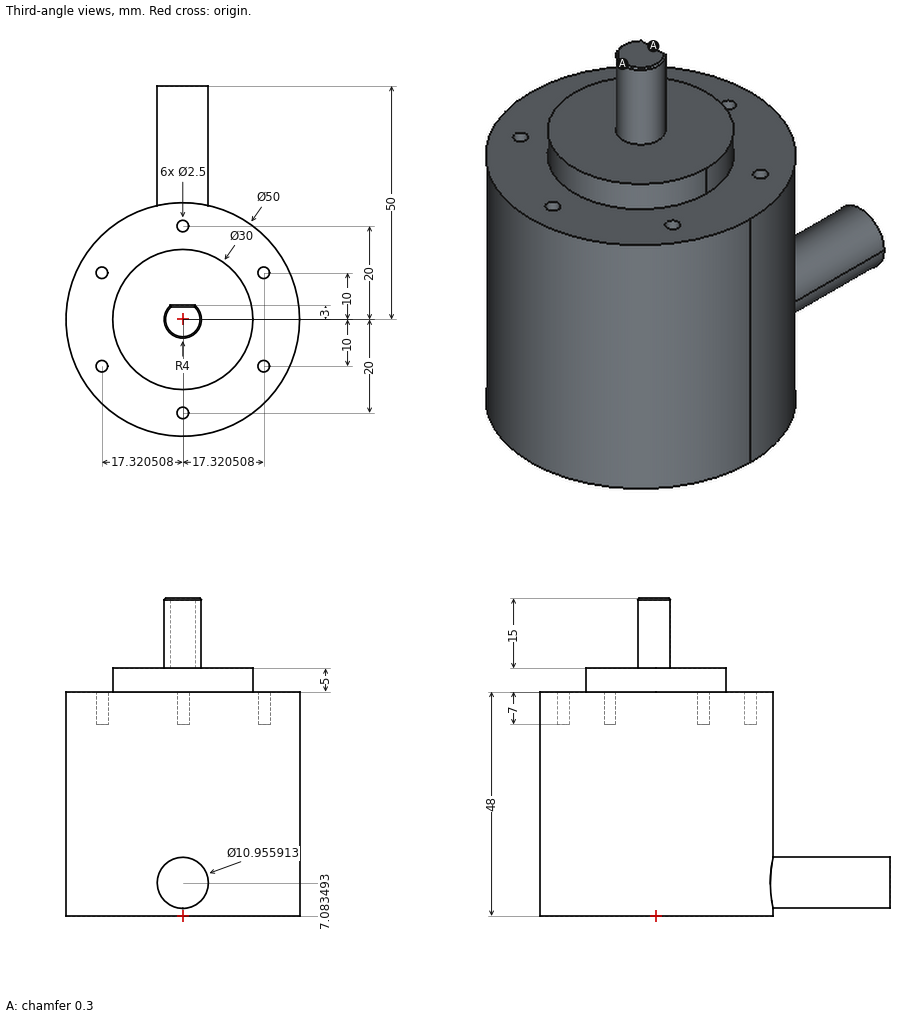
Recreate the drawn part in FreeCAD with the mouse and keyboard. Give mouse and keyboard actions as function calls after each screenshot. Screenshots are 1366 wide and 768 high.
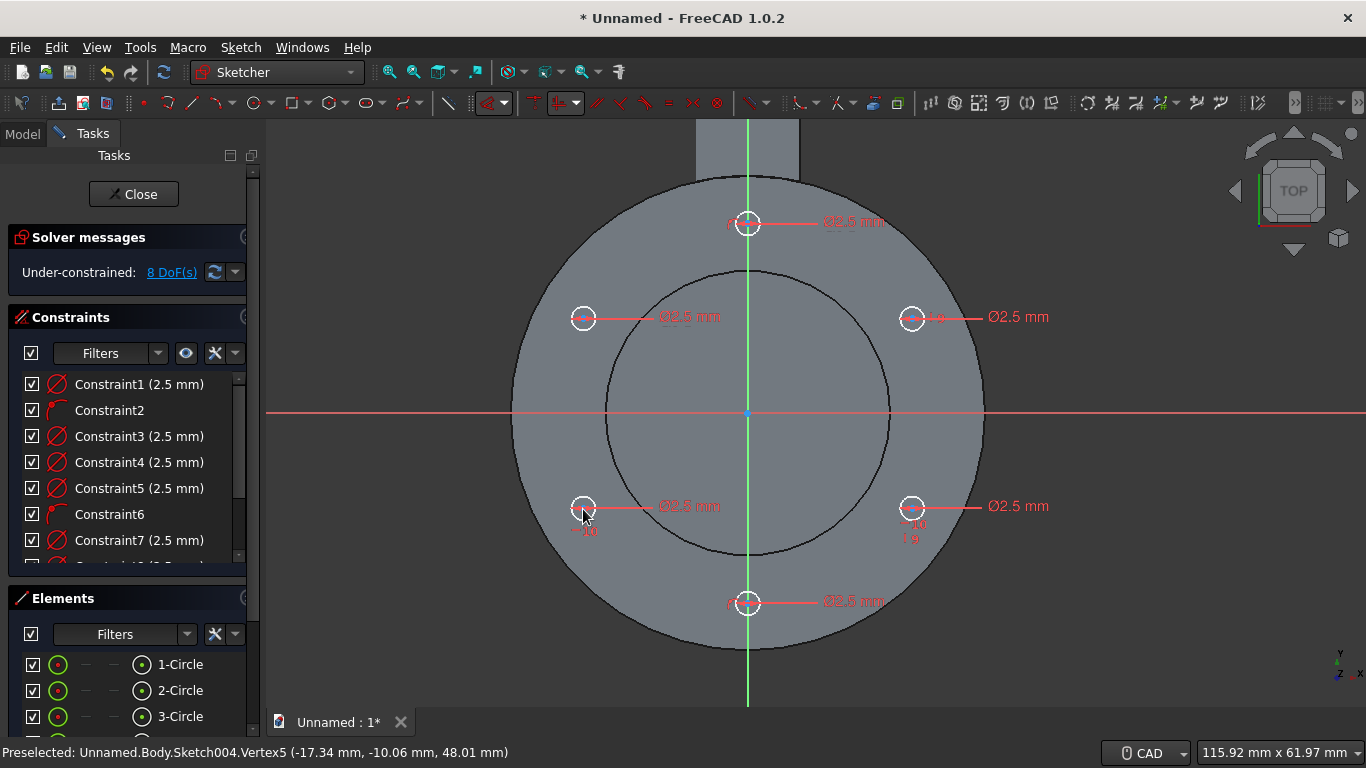
click(583, 508)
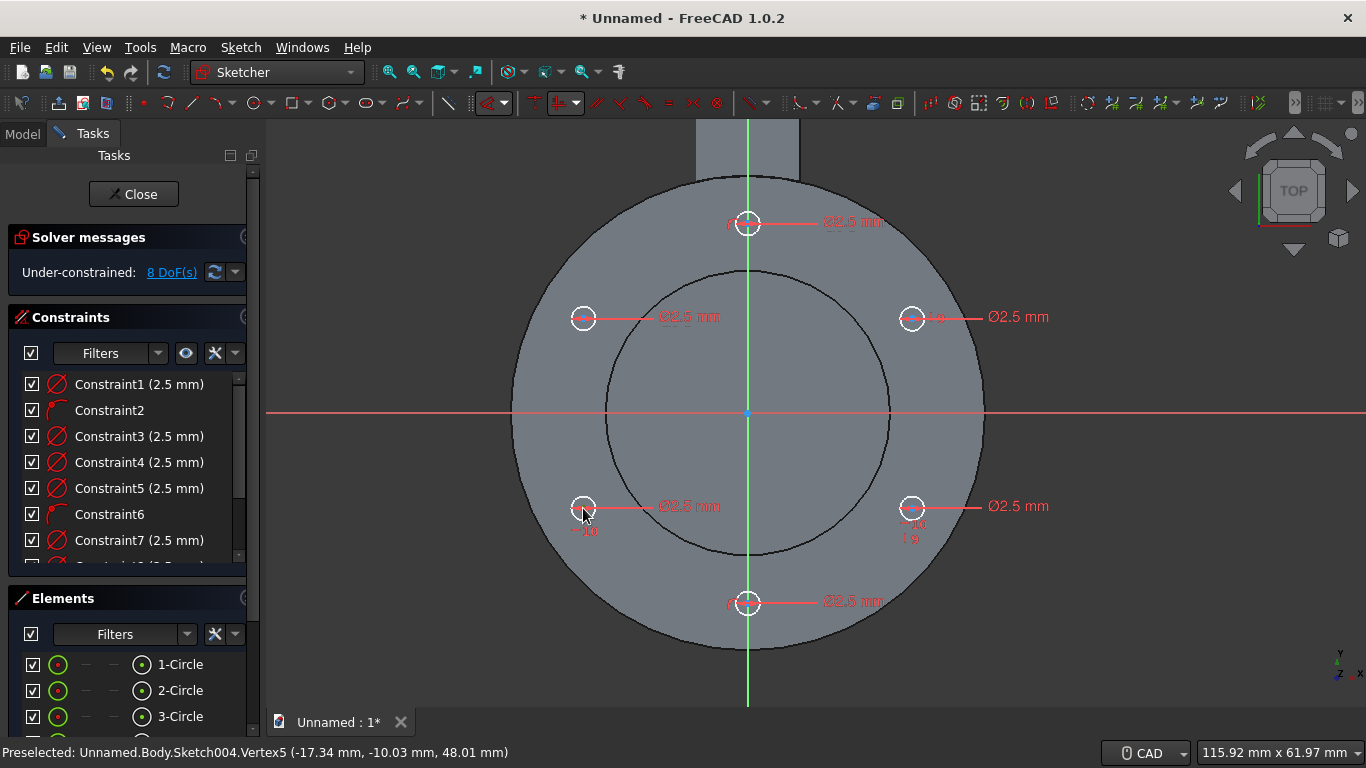
click(584, 319)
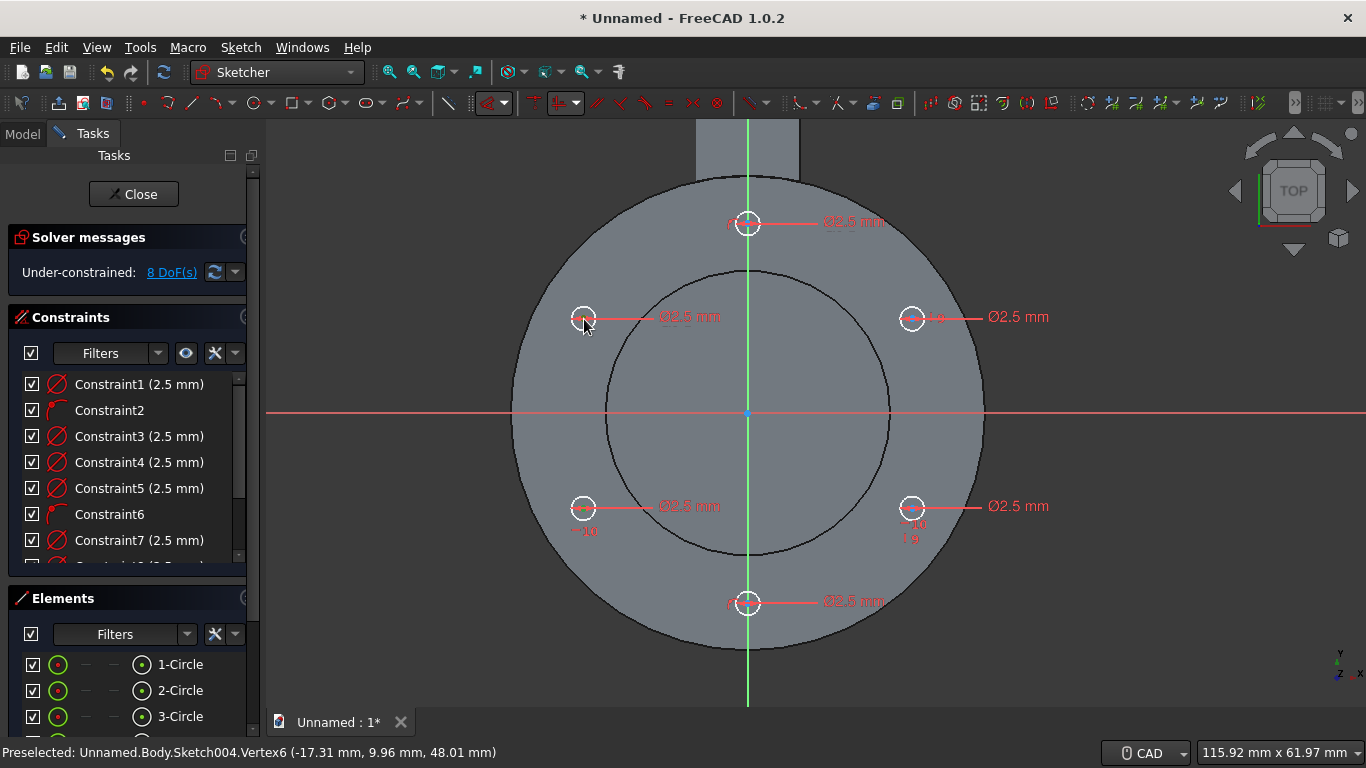
click(578, 104)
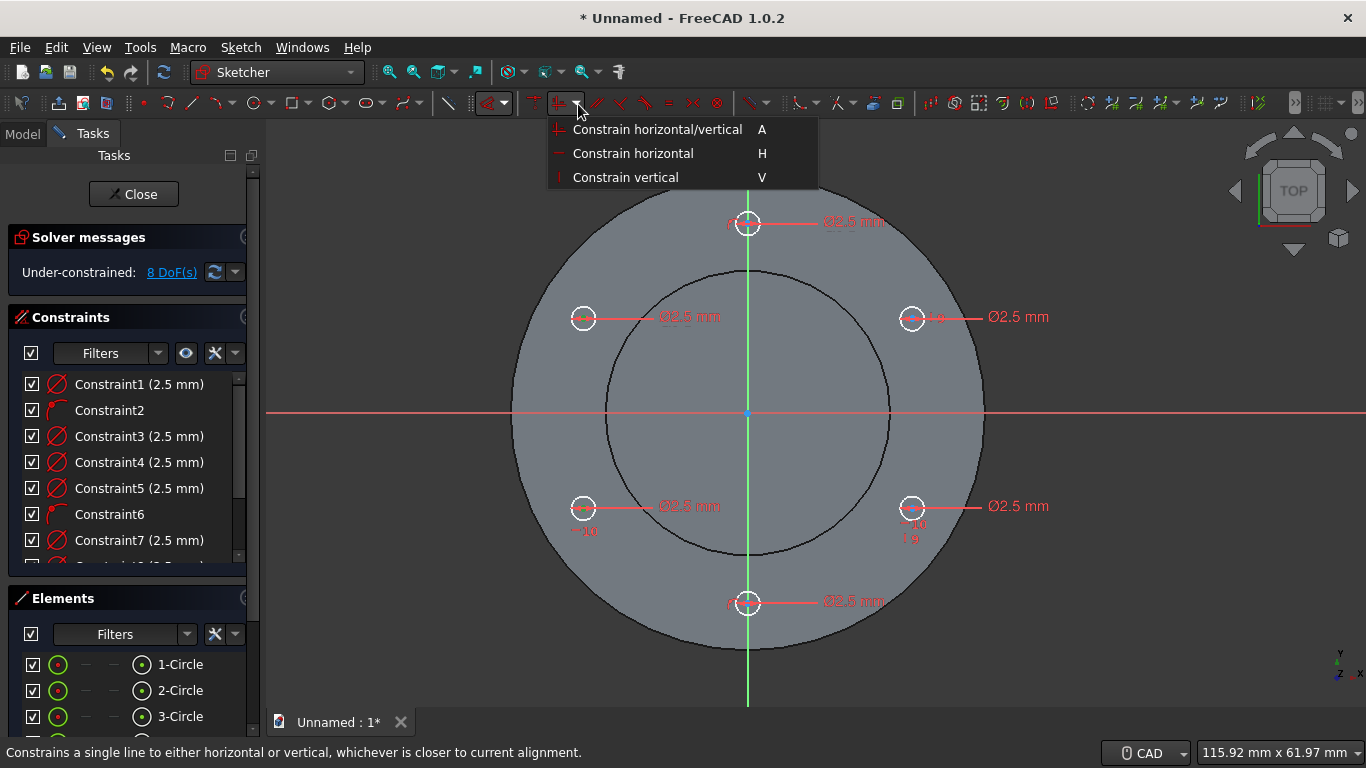
click(683, 177)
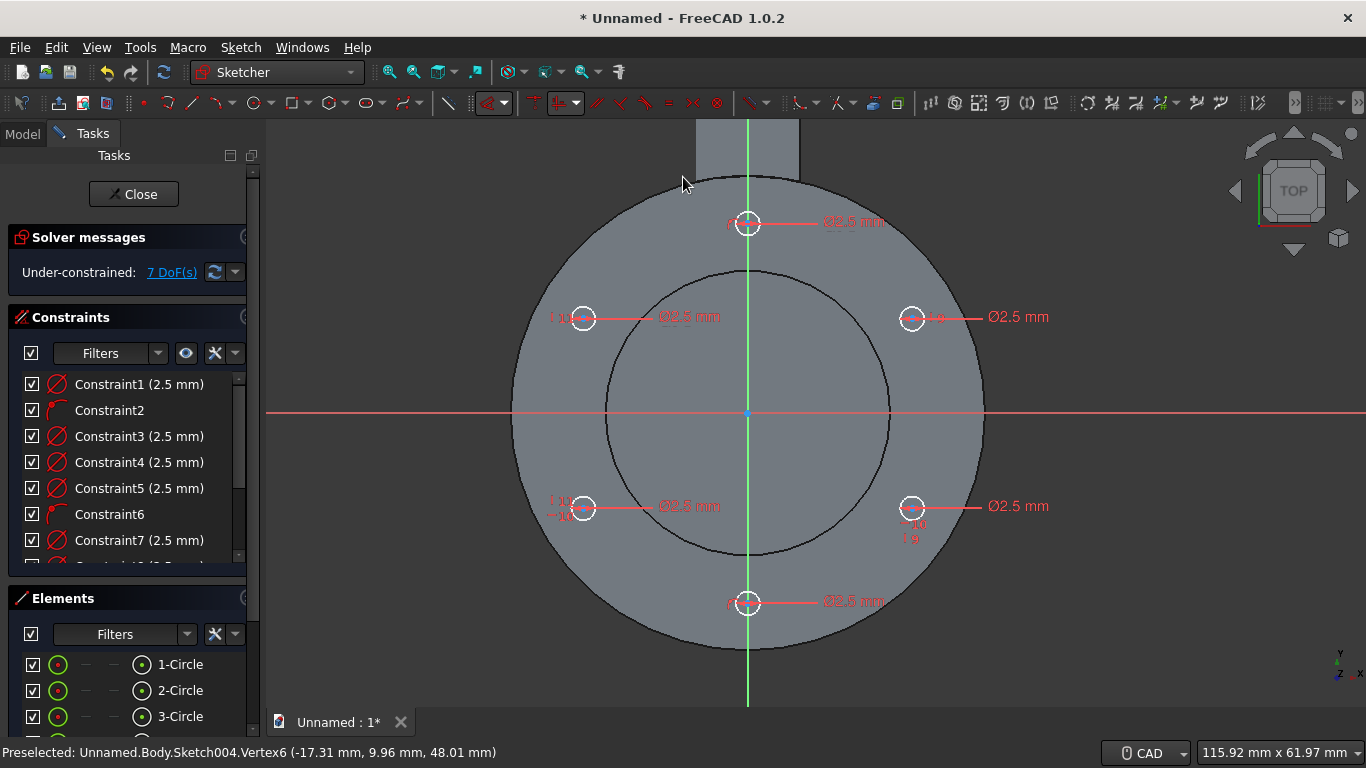
click(912, 319)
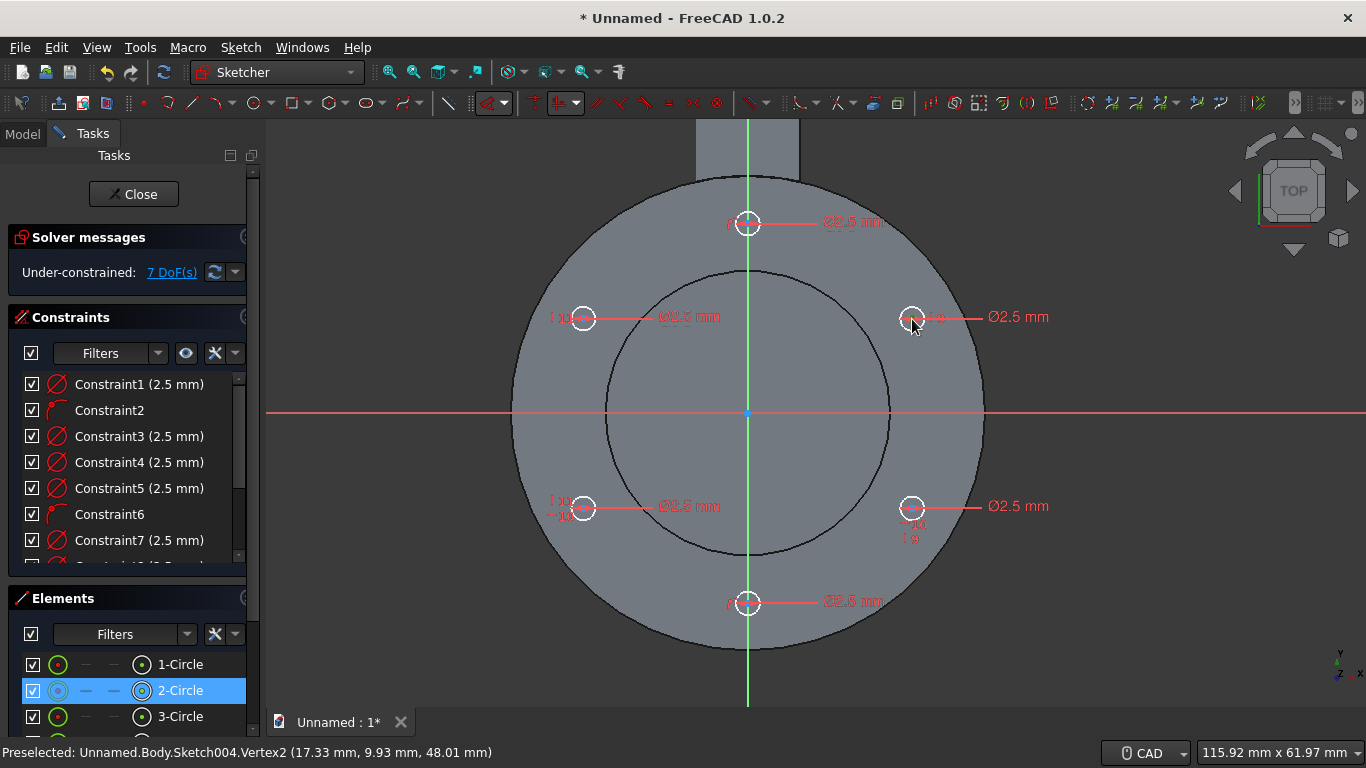
click(583, 319)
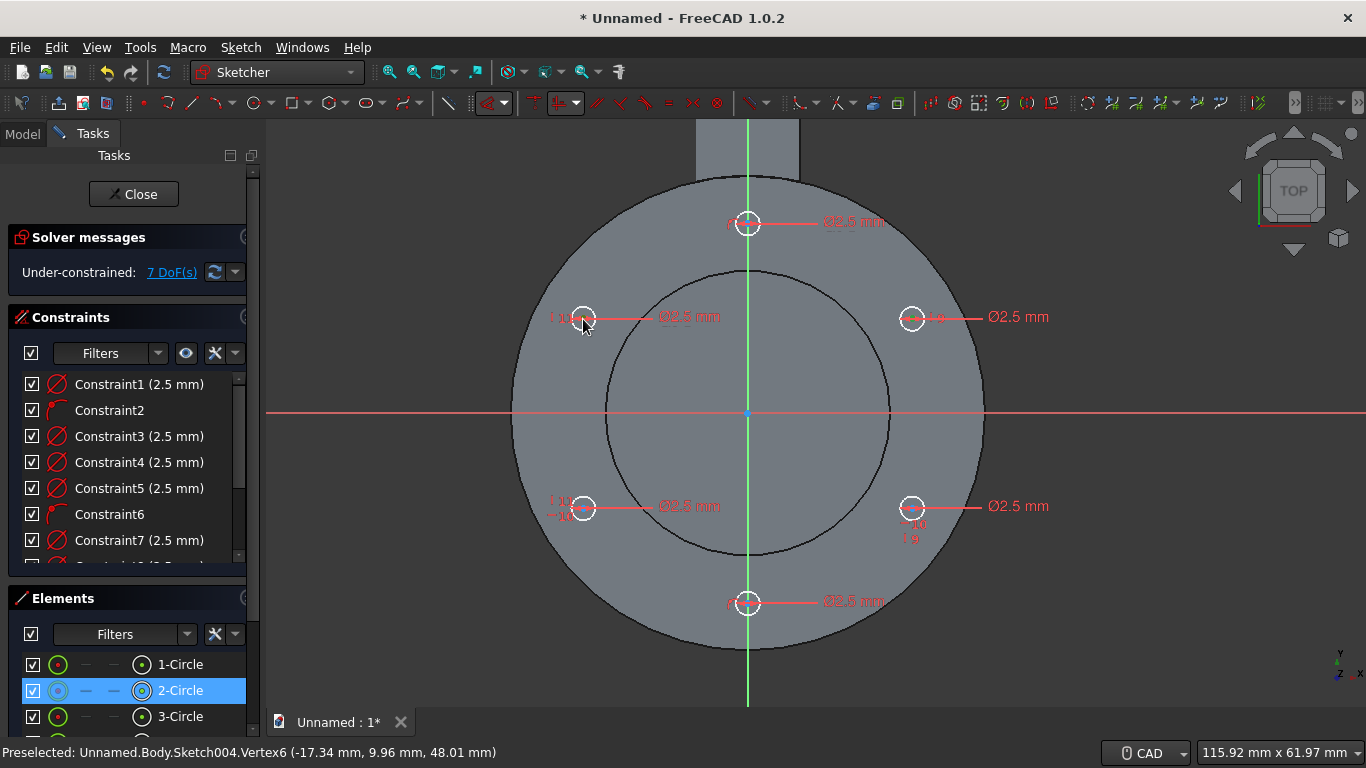
click(578, 104)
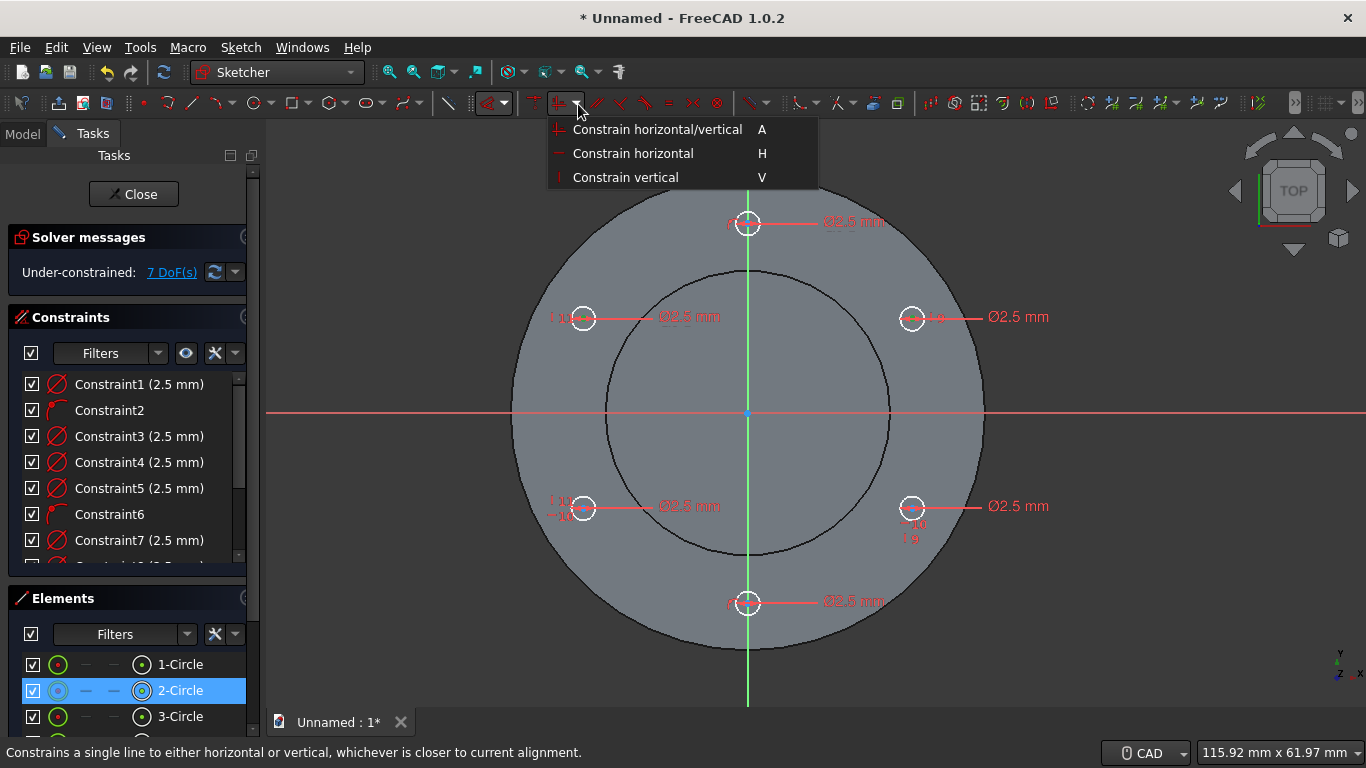
click(683, 153)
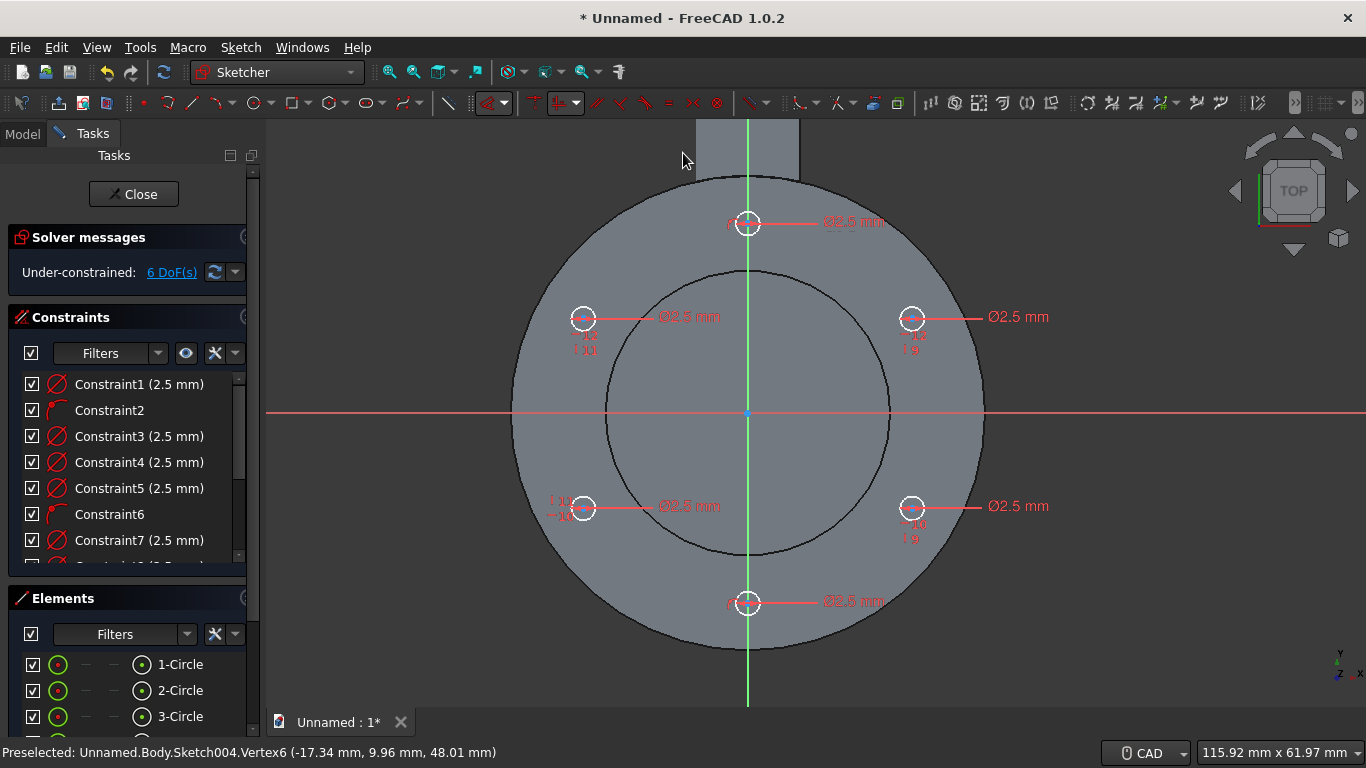
click(748, 224)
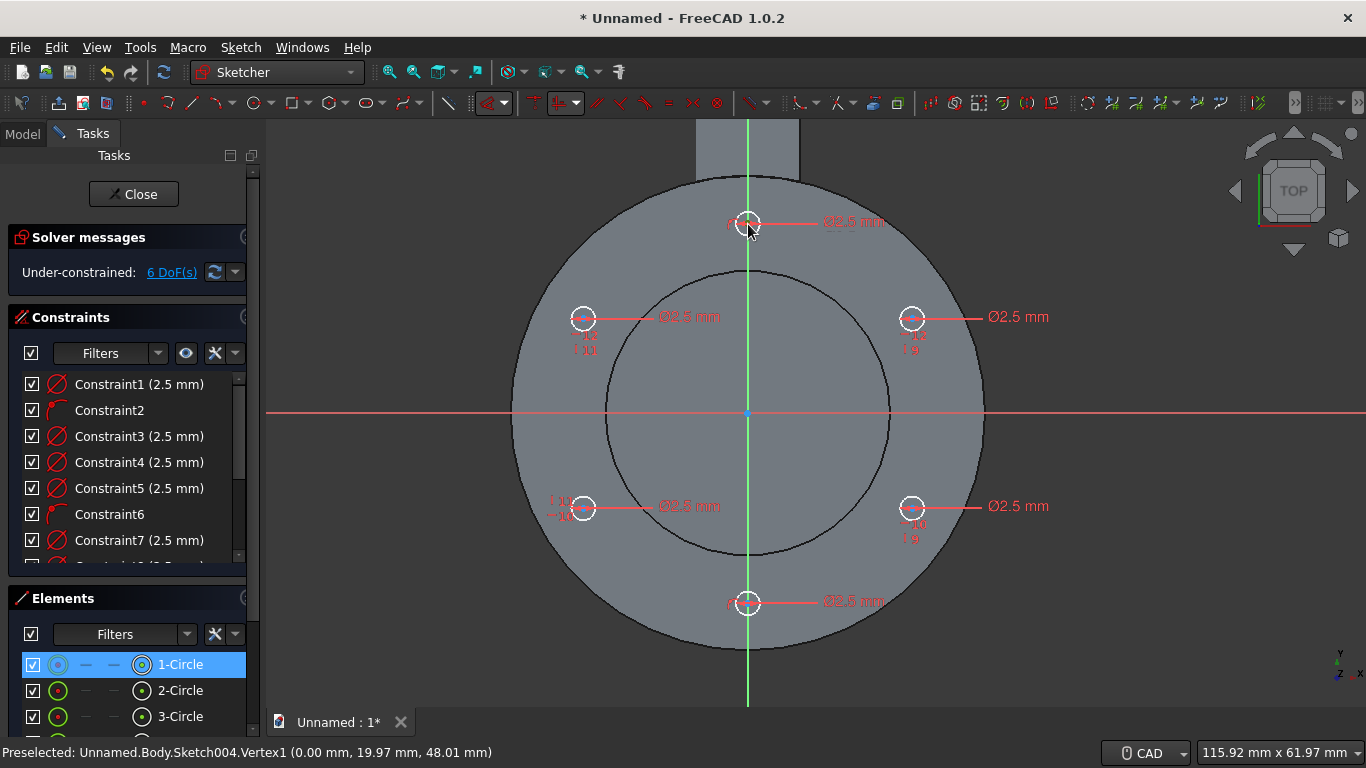
key(i)